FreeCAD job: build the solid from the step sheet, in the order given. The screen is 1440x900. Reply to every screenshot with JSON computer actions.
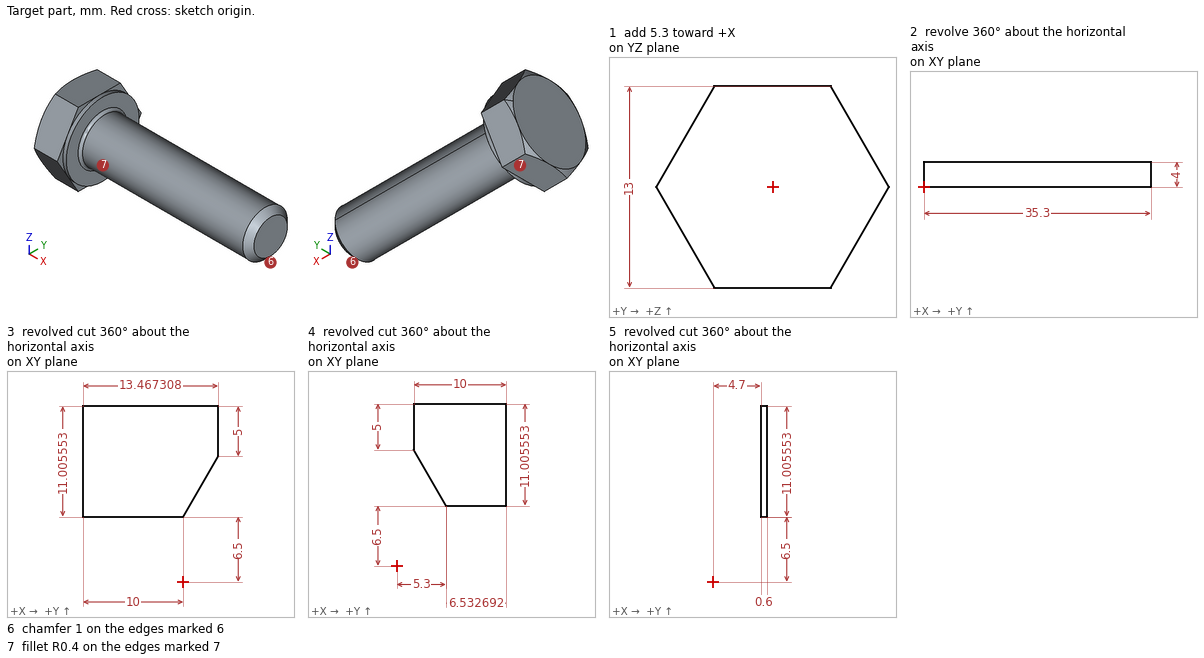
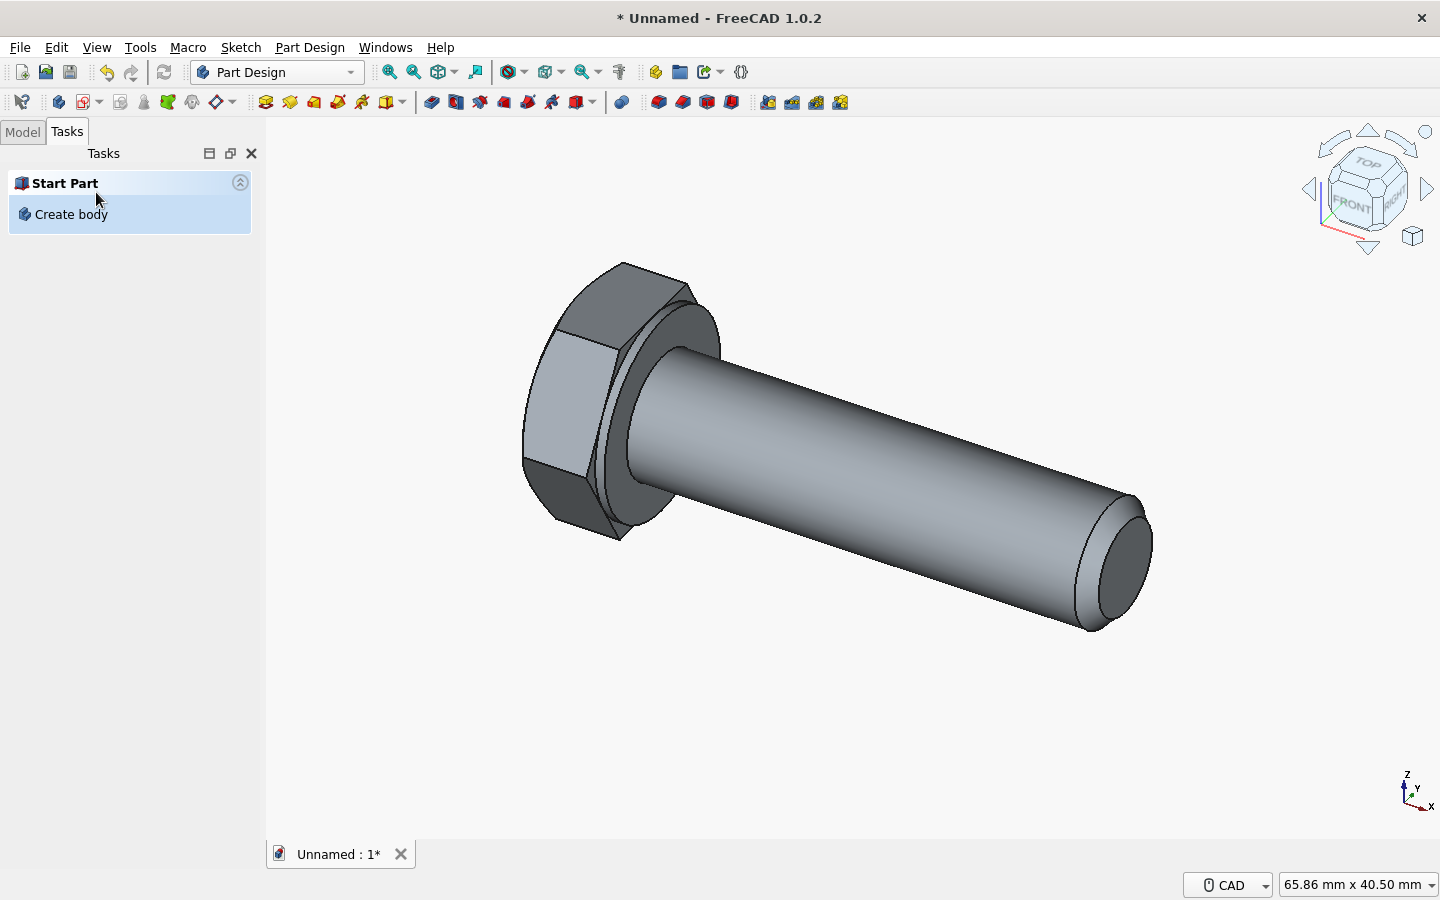
{"action": "key", "text": "0"}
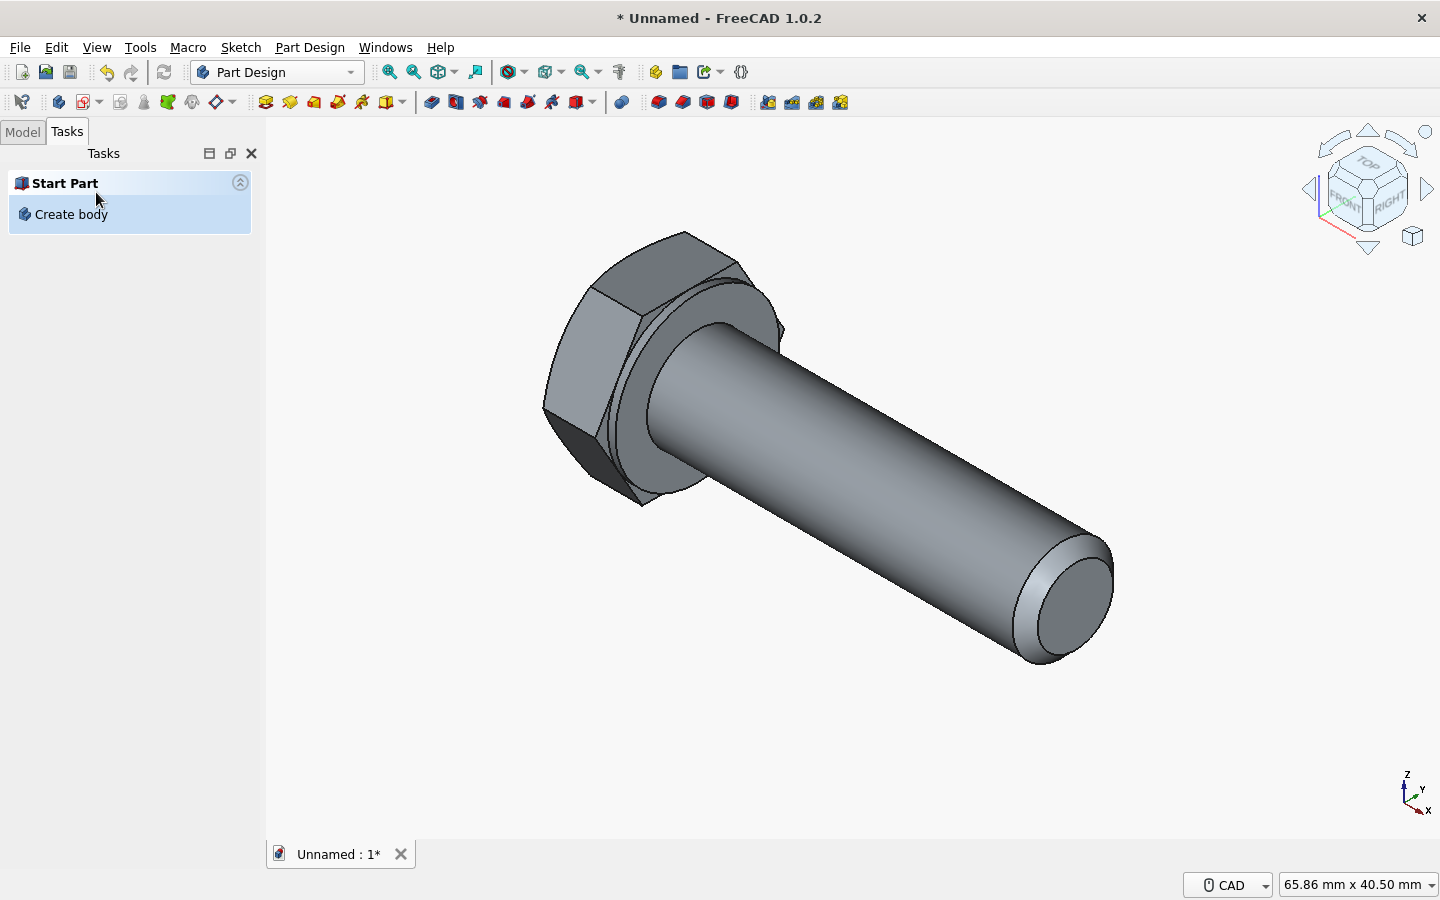
{"action": "key", "text": "2"}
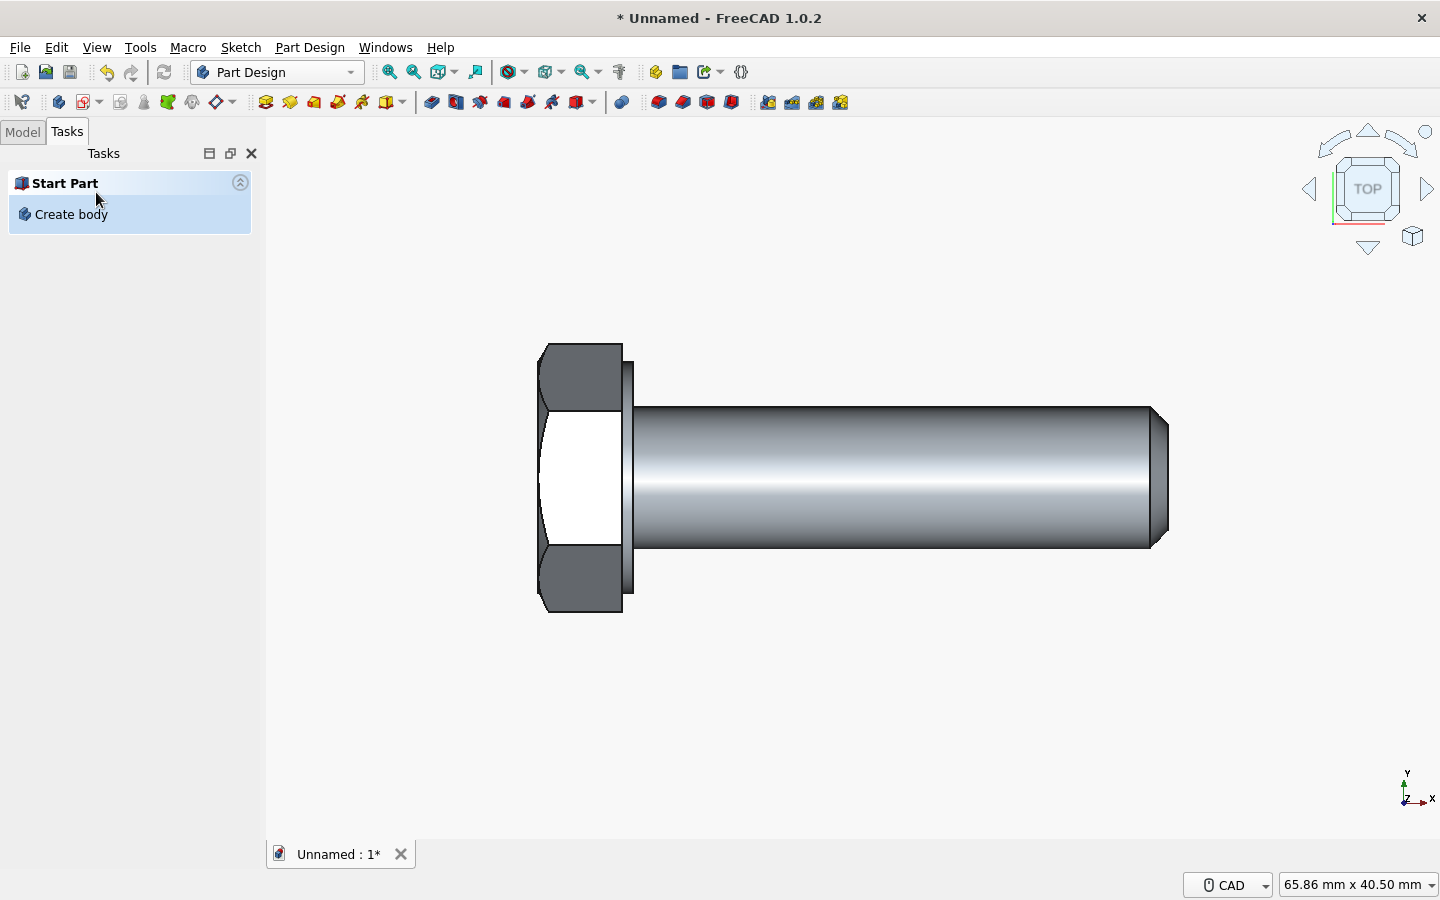
{"action": "key", "text": "1"}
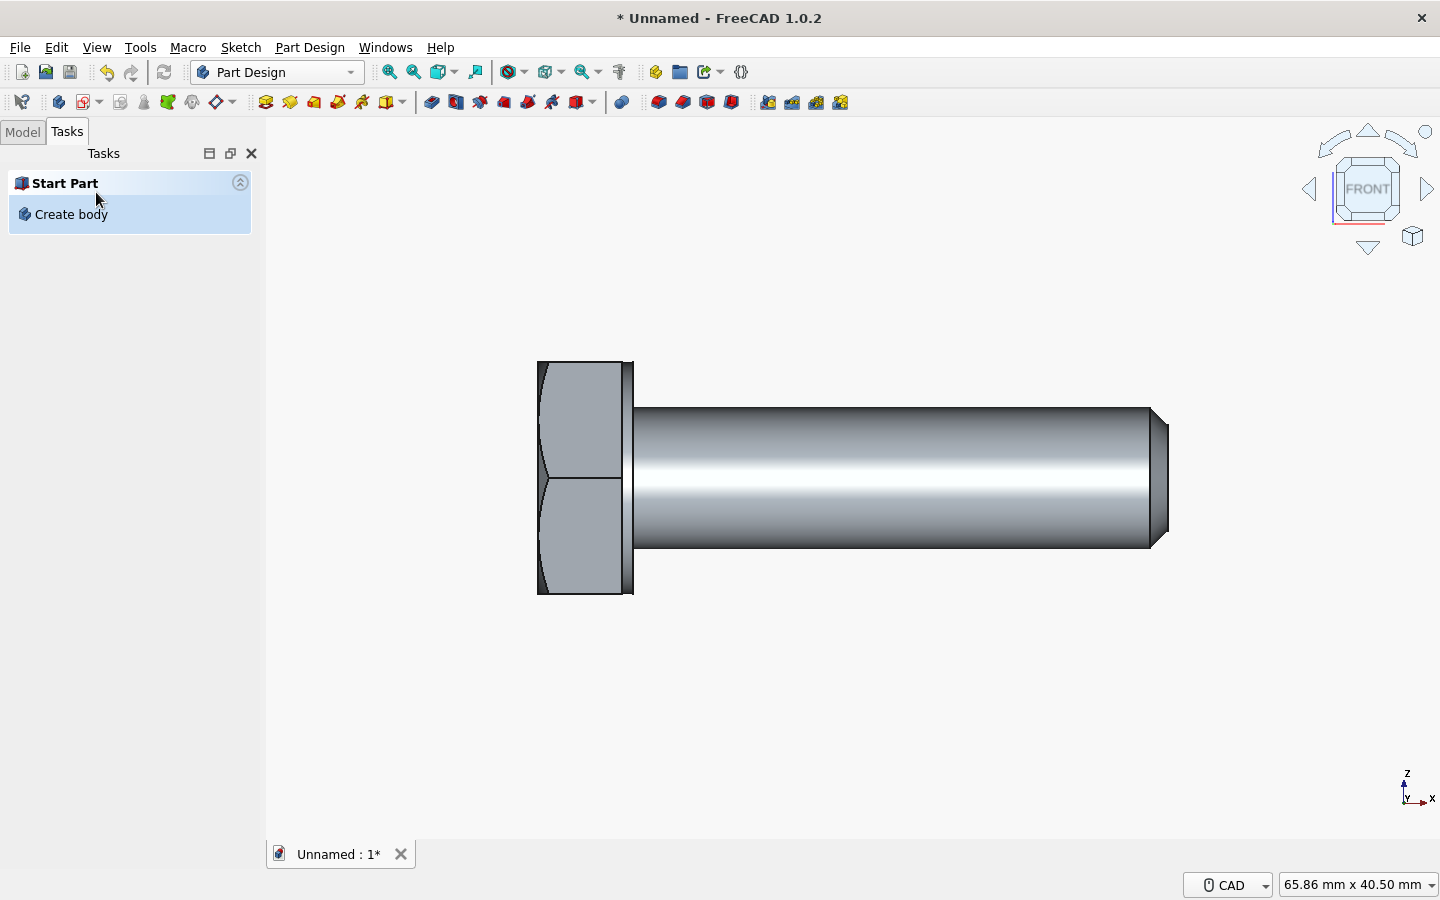
{"action": "key", "text": "3"}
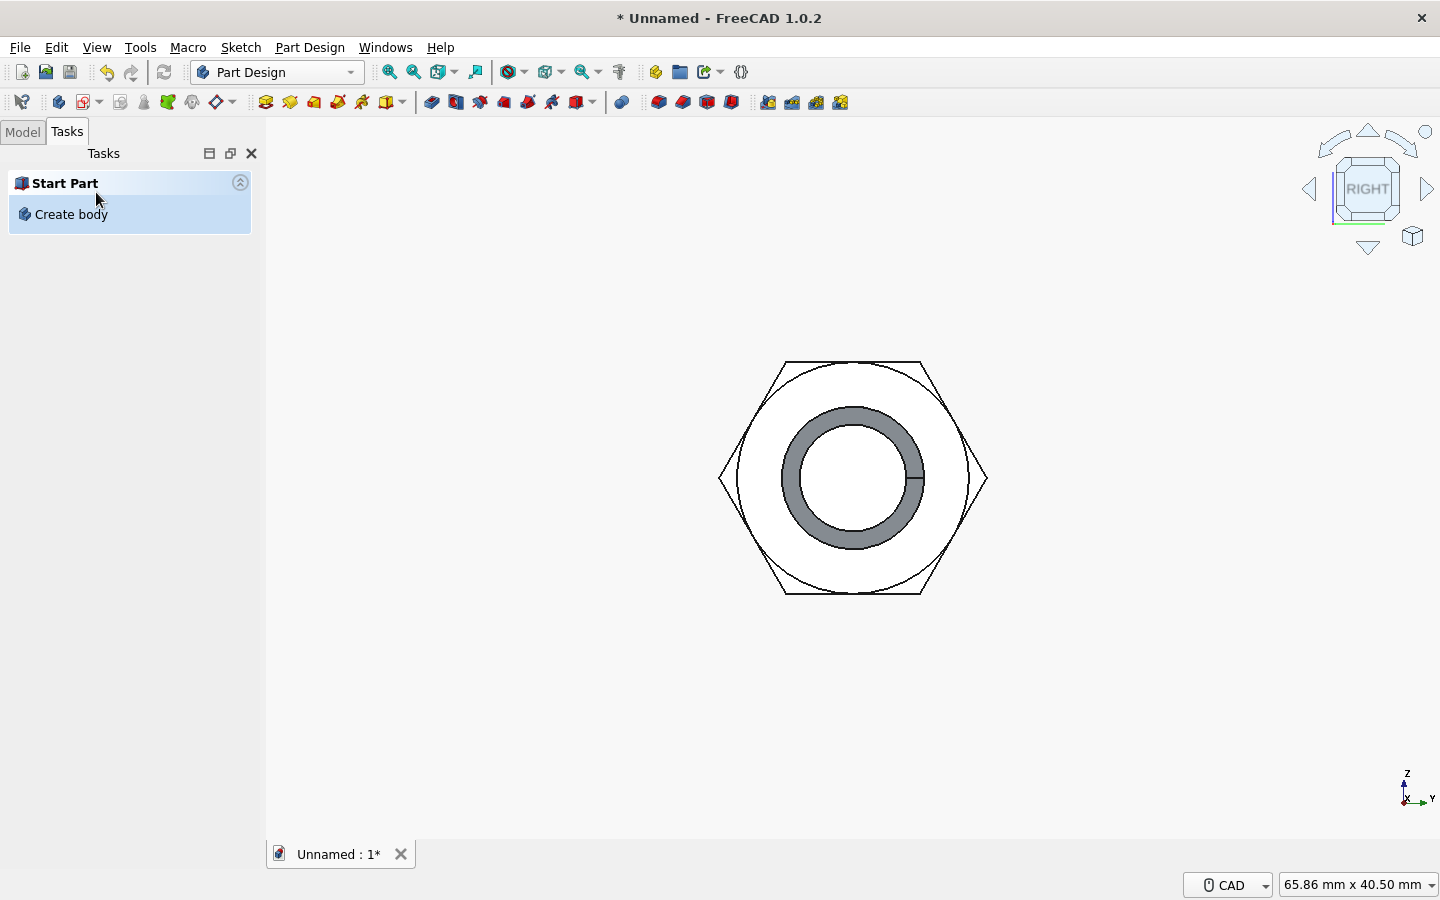
{"action": "left_click", "coordinate": [390, 72]}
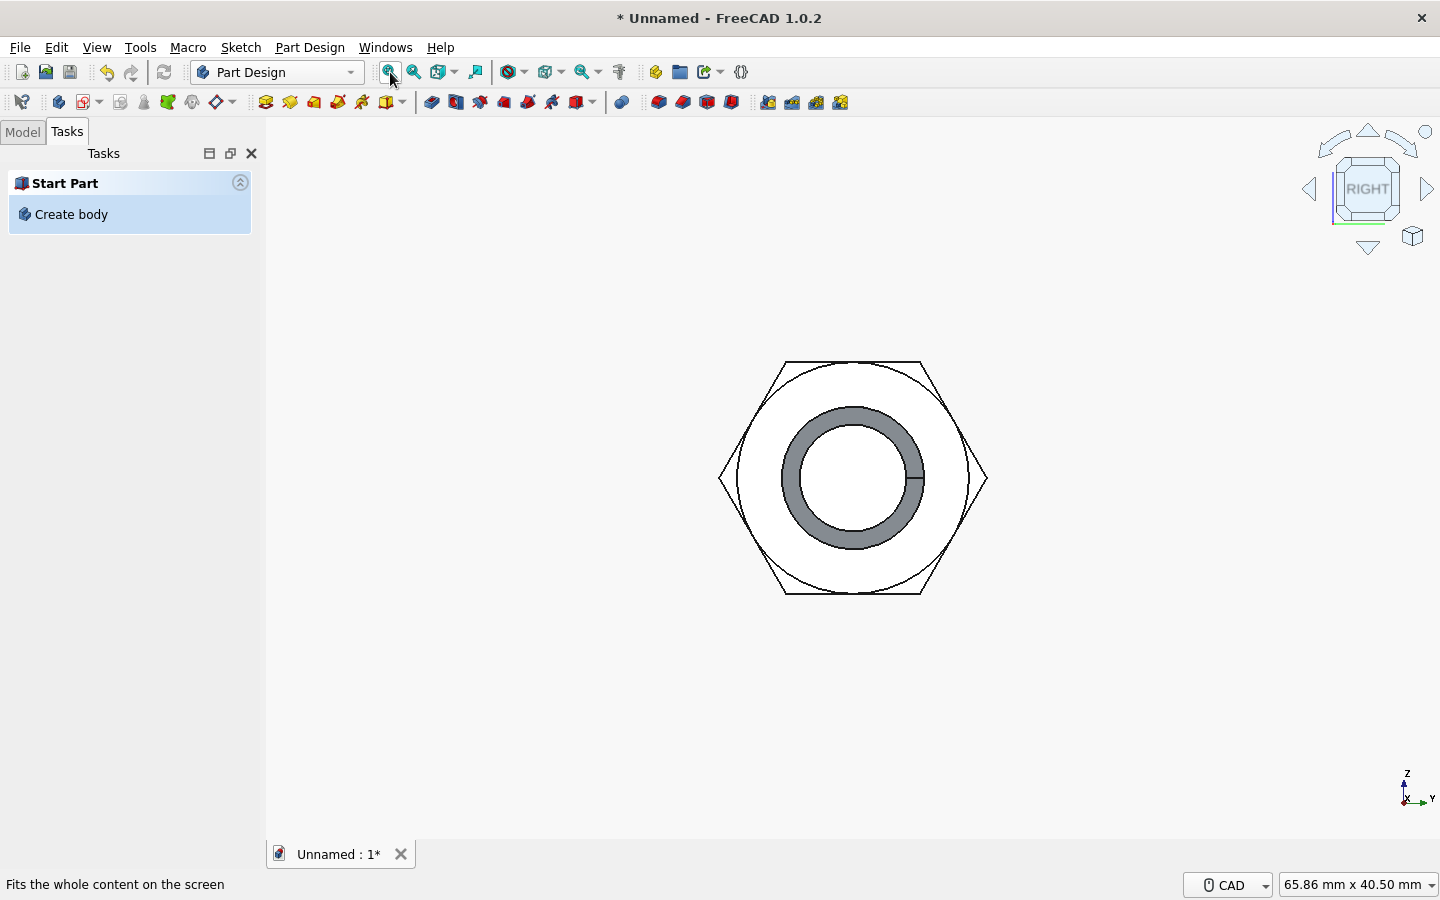
{"action": "key", "text": "5"}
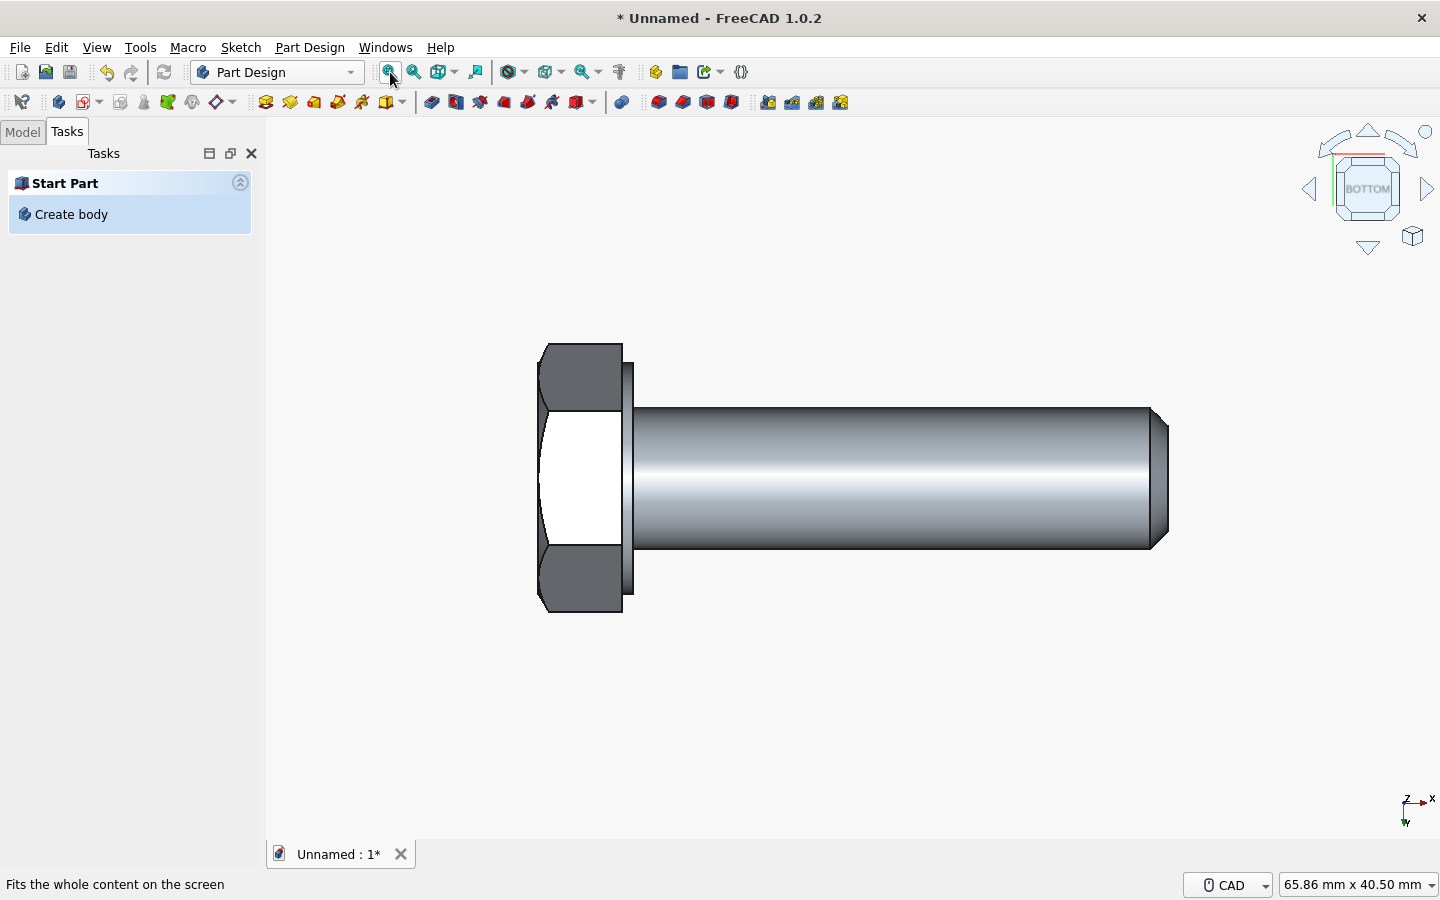
{"action": "key", "text": "4"}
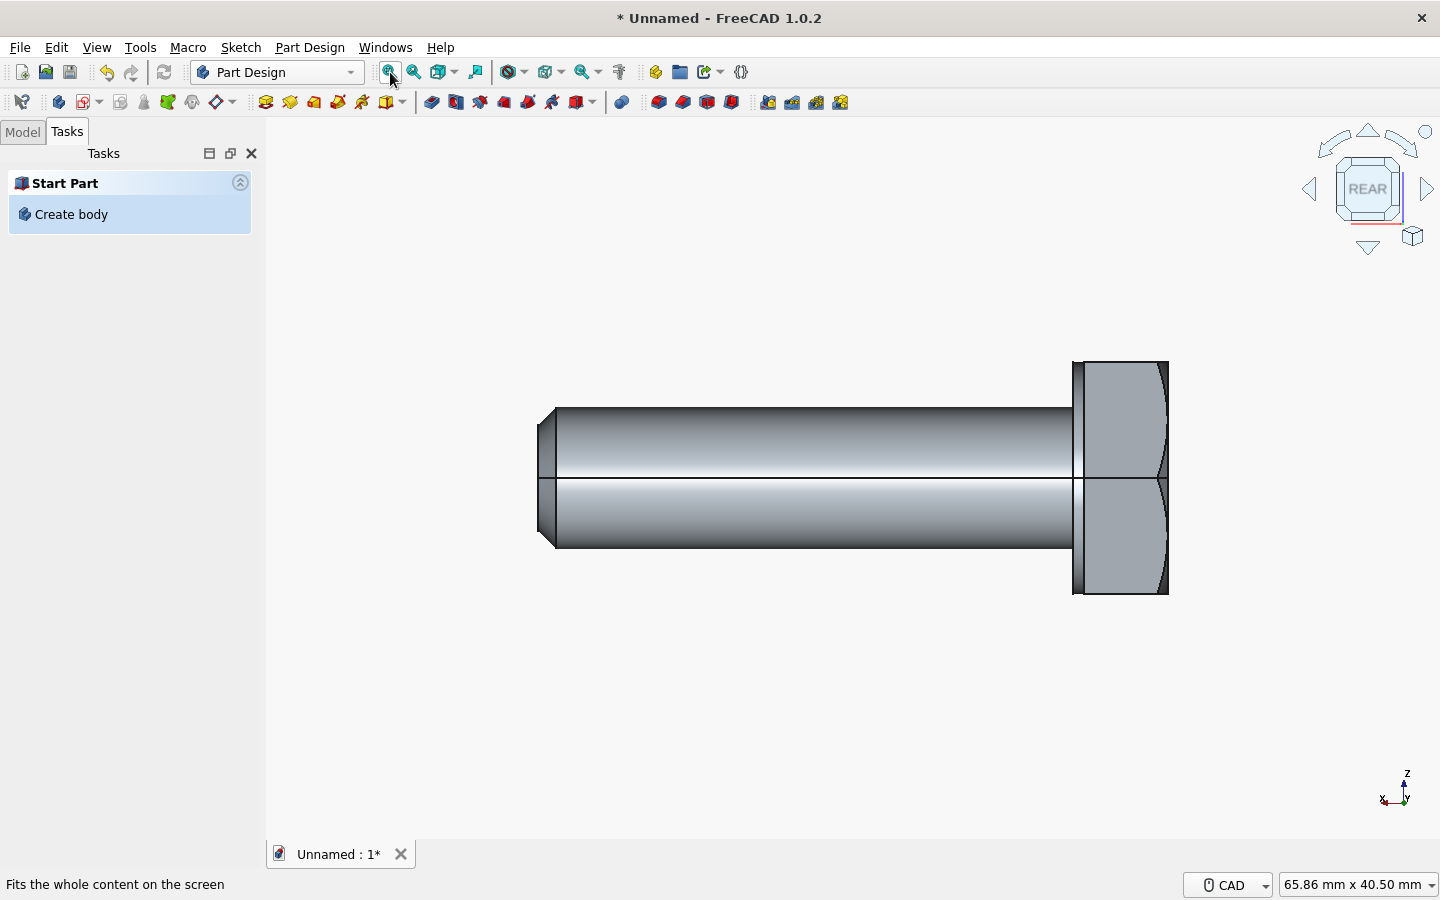
{"action": "key", "text": "6"}